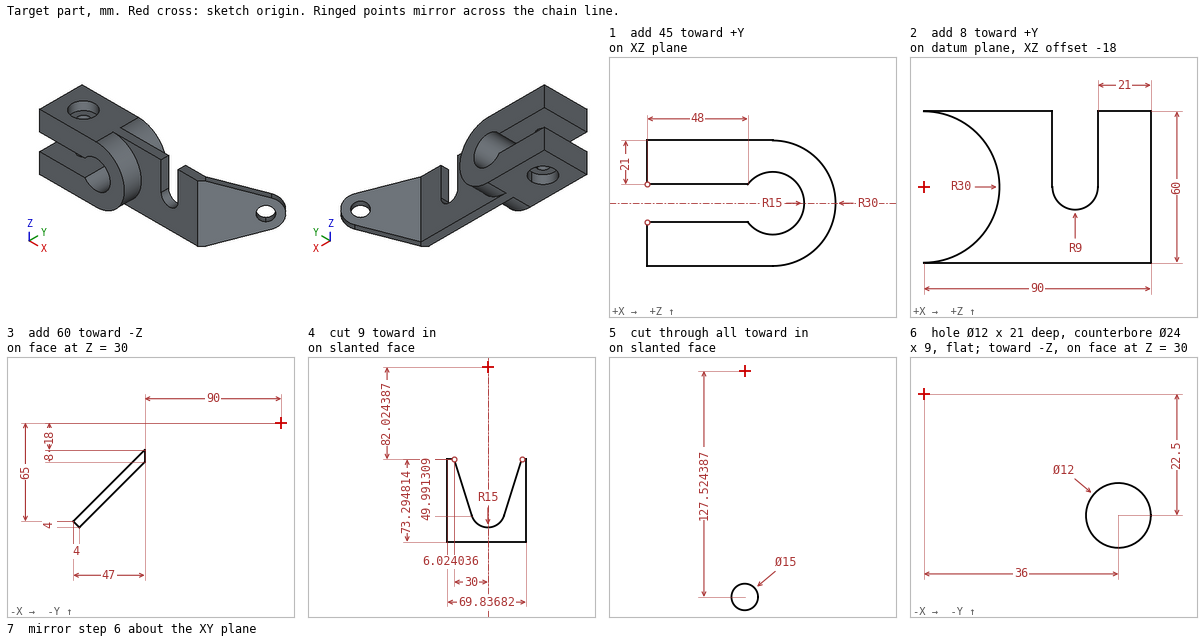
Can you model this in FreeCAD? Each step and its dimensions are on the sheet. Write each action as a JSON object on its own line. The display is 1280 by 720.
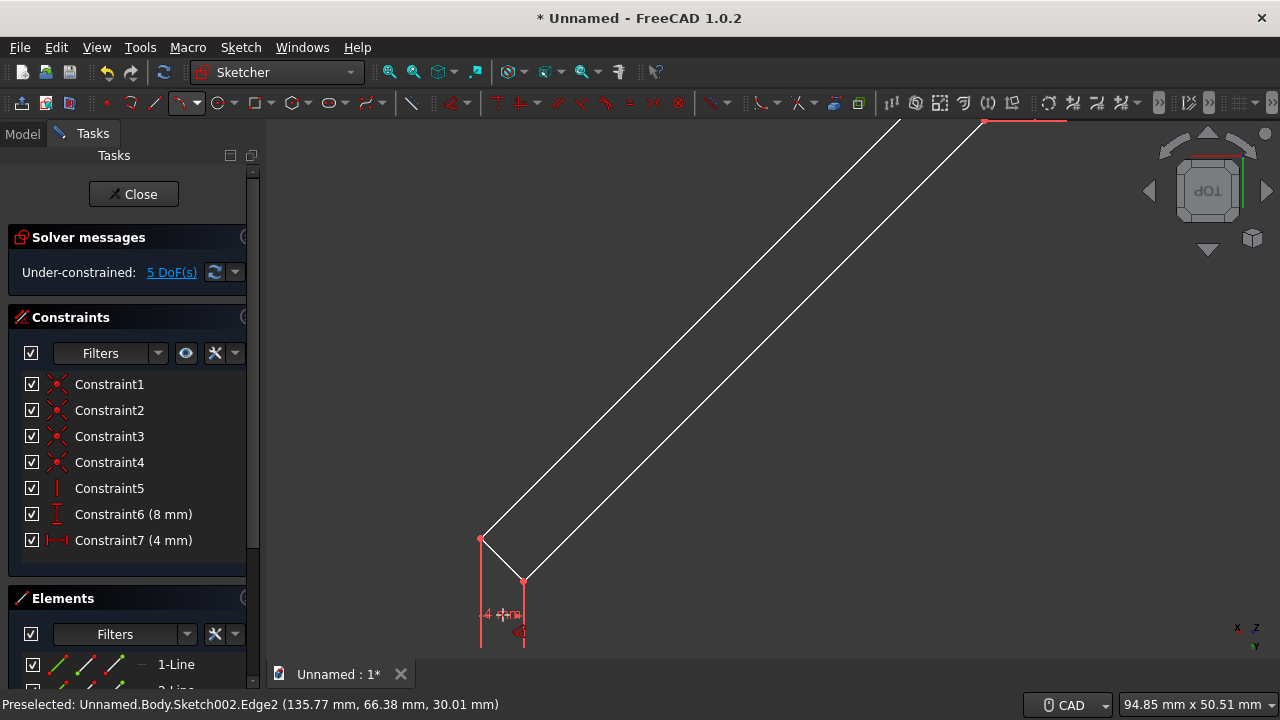
{"action": "left_click", "coordinate": [494, 551]}
{"action": "left_click", "coordinate": [447, 560]}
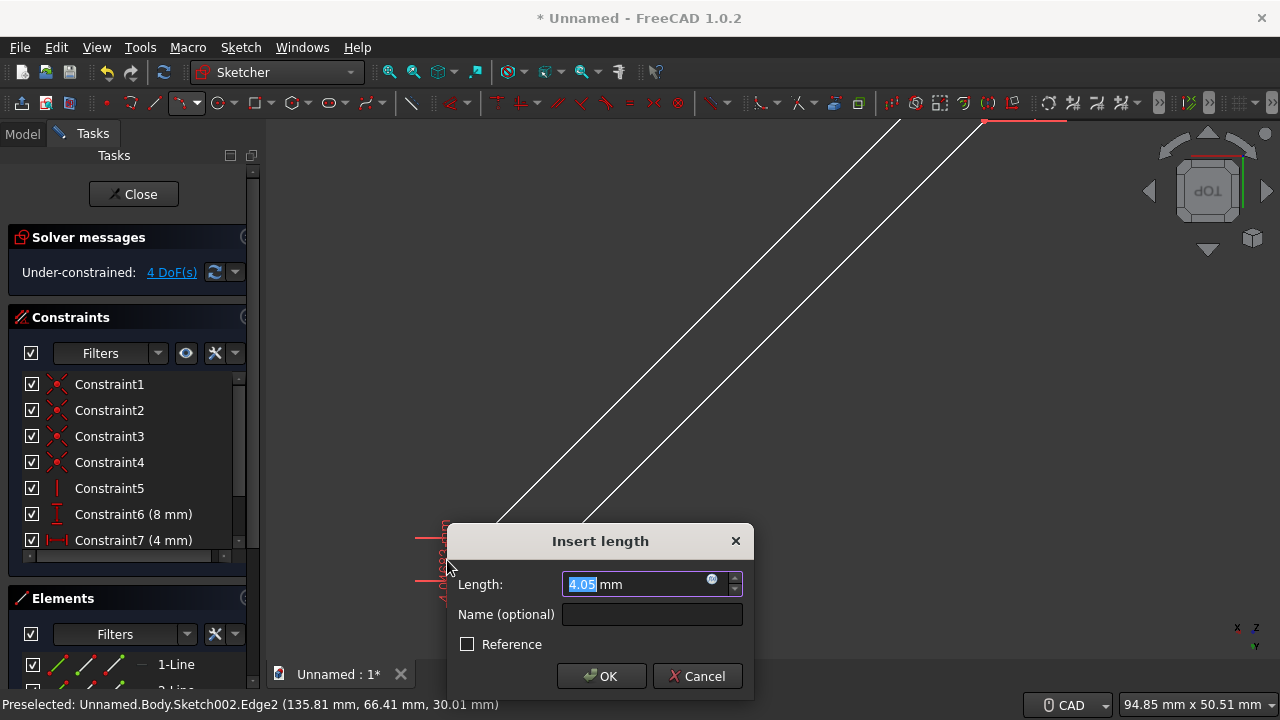
{"action": "type", "text": "4"}
{"action": "key", "text": "Return"}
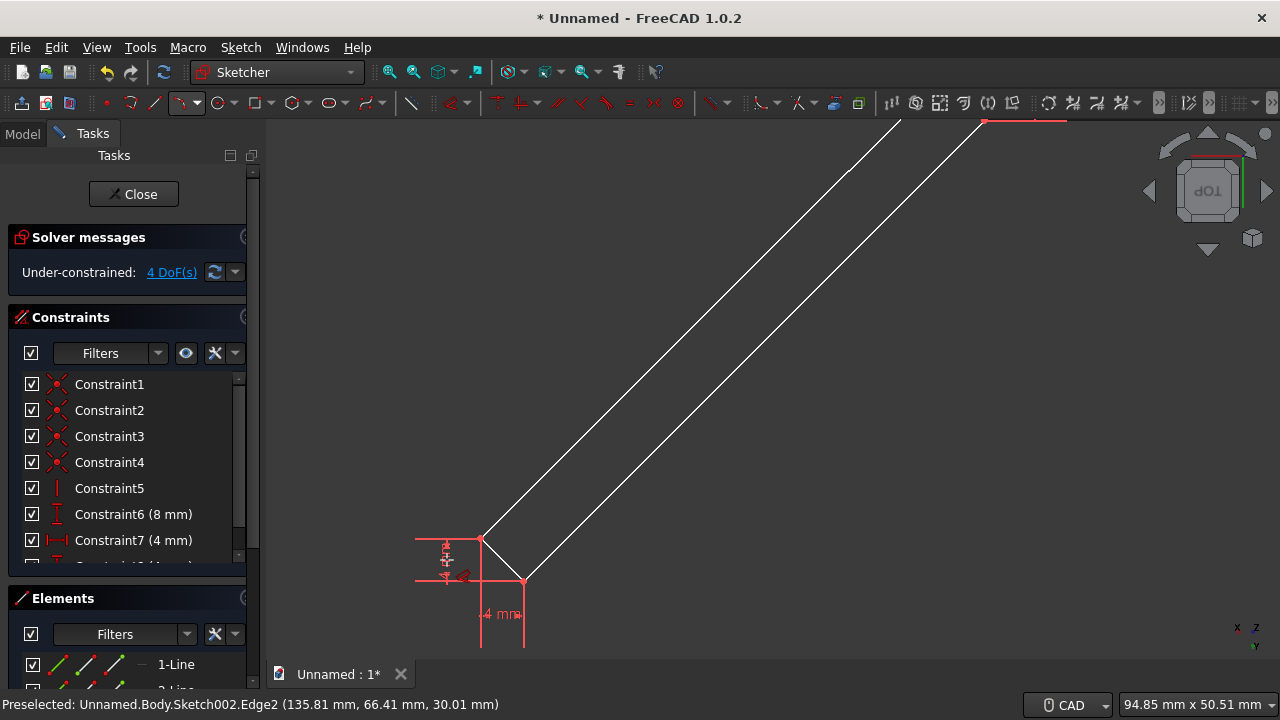
{"action": "scroll", "coordinate": [647, 556], "scroll_direction": "down", "scroll_amount": 2}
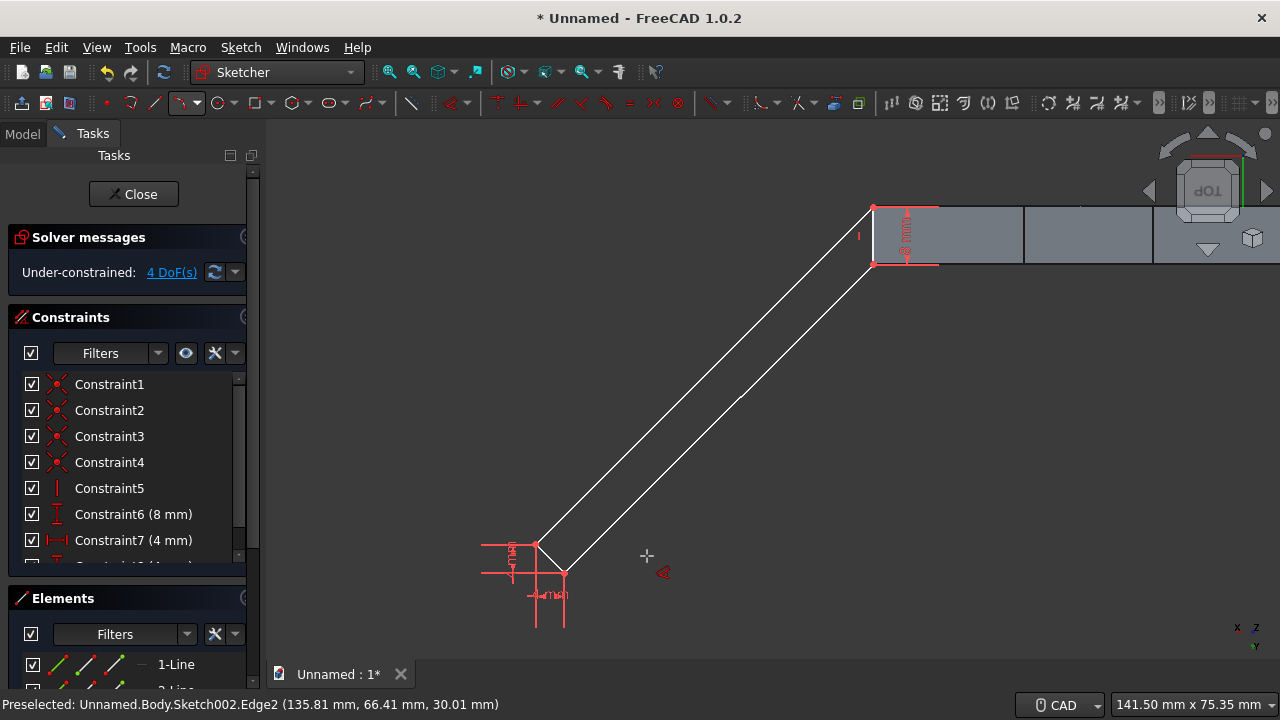
{"action": "left_click", "coordinate": [873, 207]}
{"action": "left_click", "coordinate": [994, 241]}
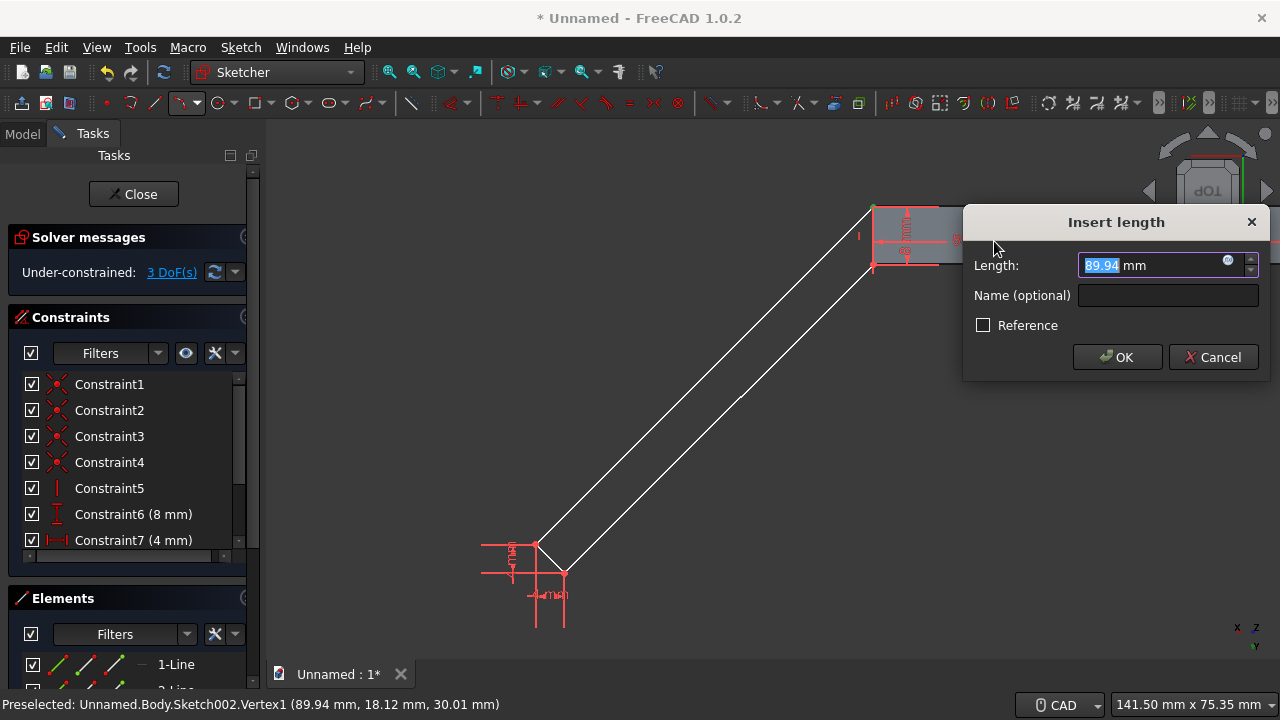
{"action": "type", "text": "90"}
{"action": "key", "text": "Return"}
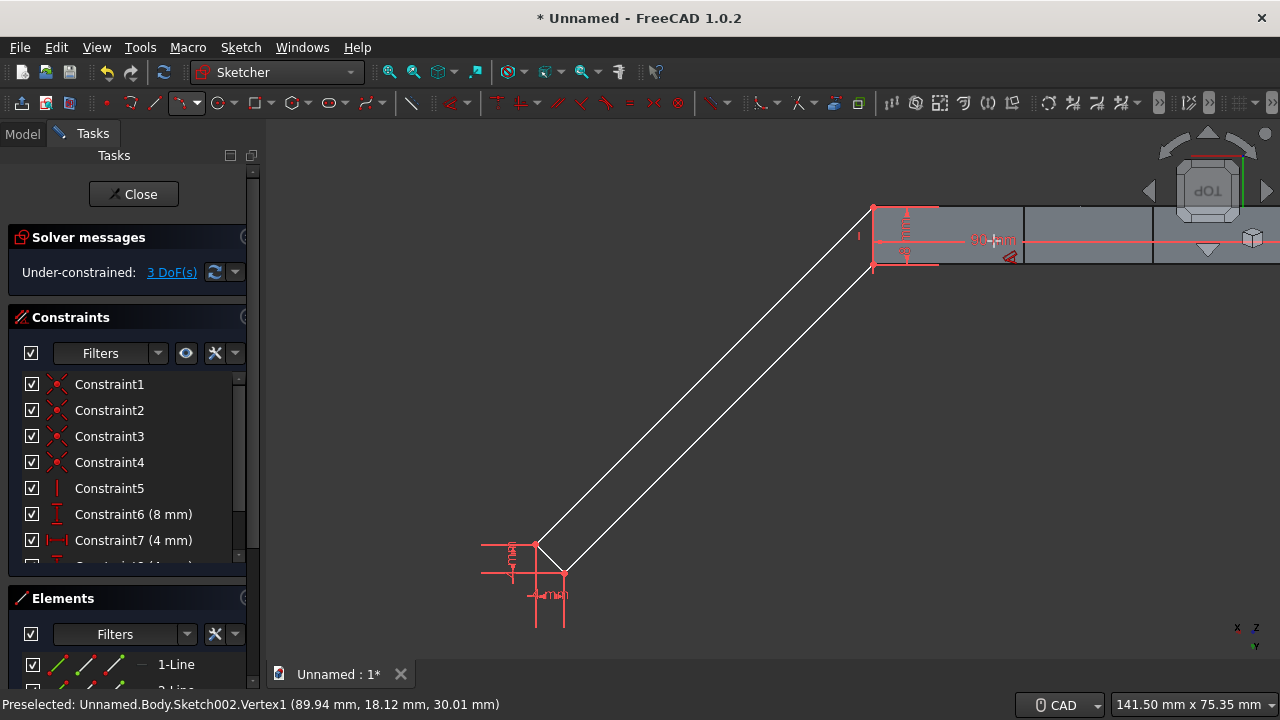
{"action": "left_click", "coordinate": [873, 207]}
{"action": "left_click", "coordinate": [839, 177]}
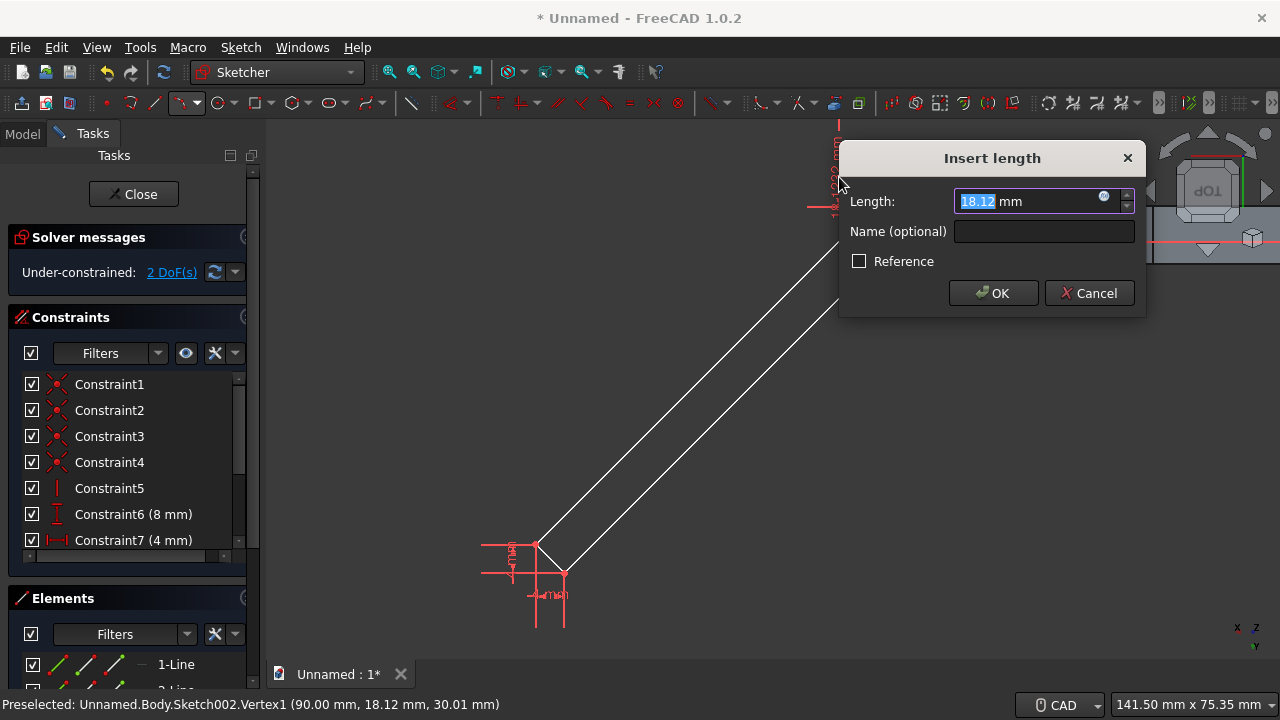
{"action": "type", "text": "18"}
{"action": "key", "text": "Return"}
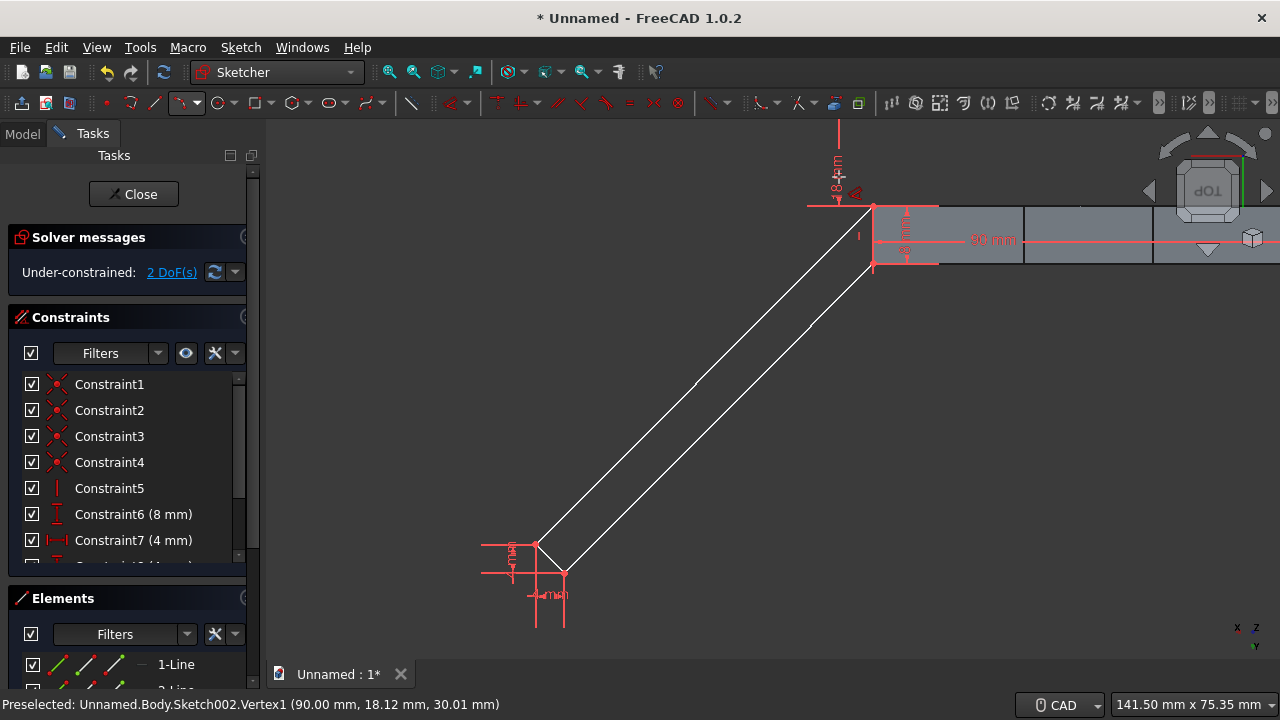
{"action": "left_click", "coordinate": [536, 545]}
{"action": "left_click", "coordinate": [502, 346]}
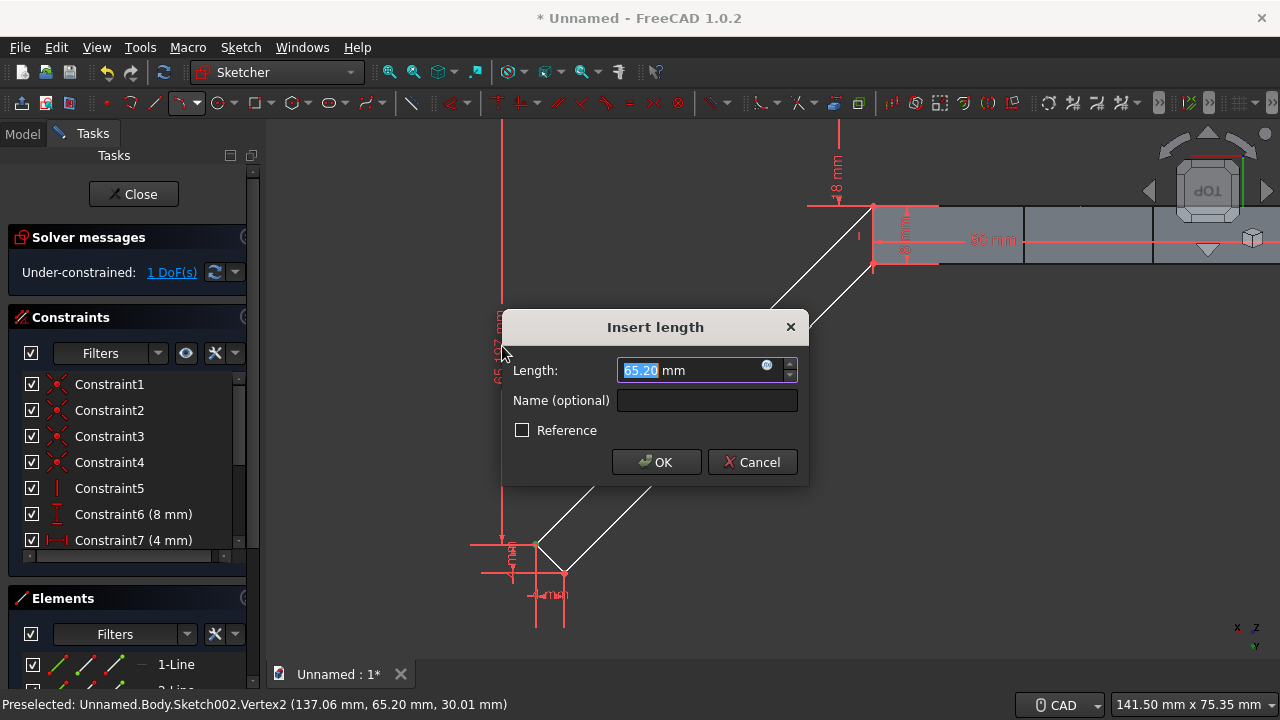
{"action": "type", "text": "65"}
{"action": "key", "text": "Return"}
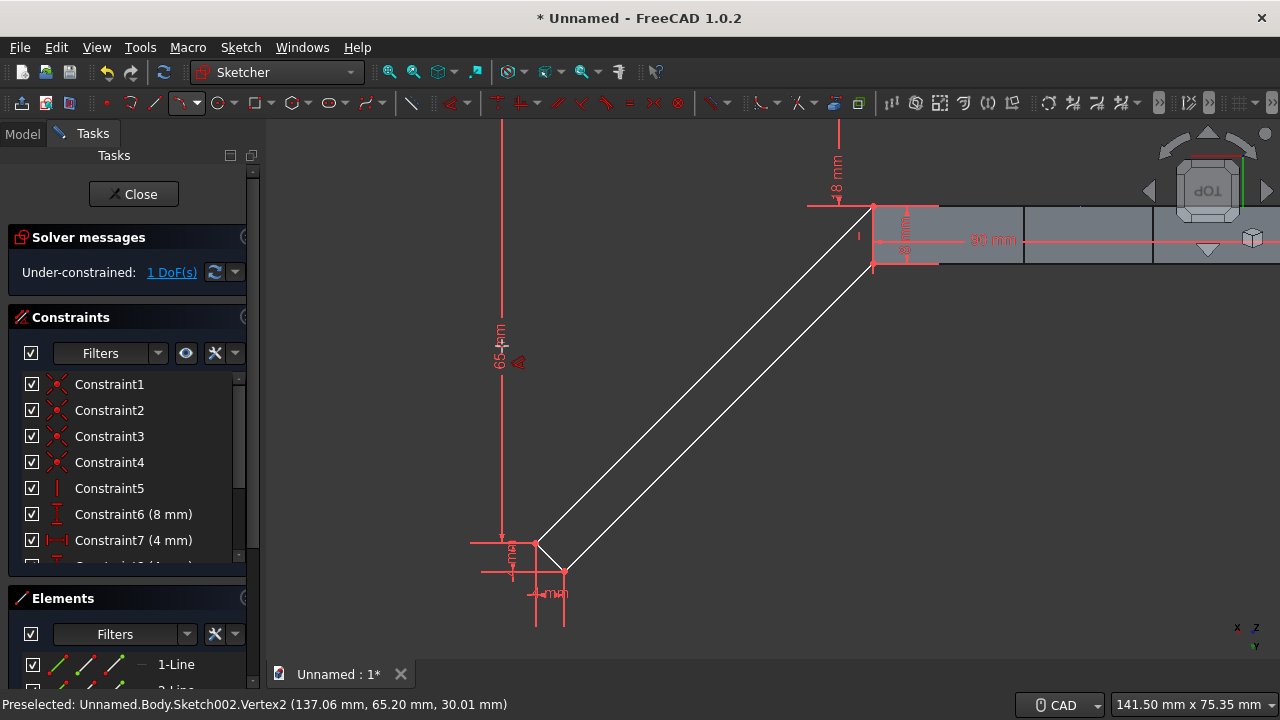
{"action": "left_click", "coordinate": [772, 307]}
{"action": "left_click", "coordinate": [704, 172]}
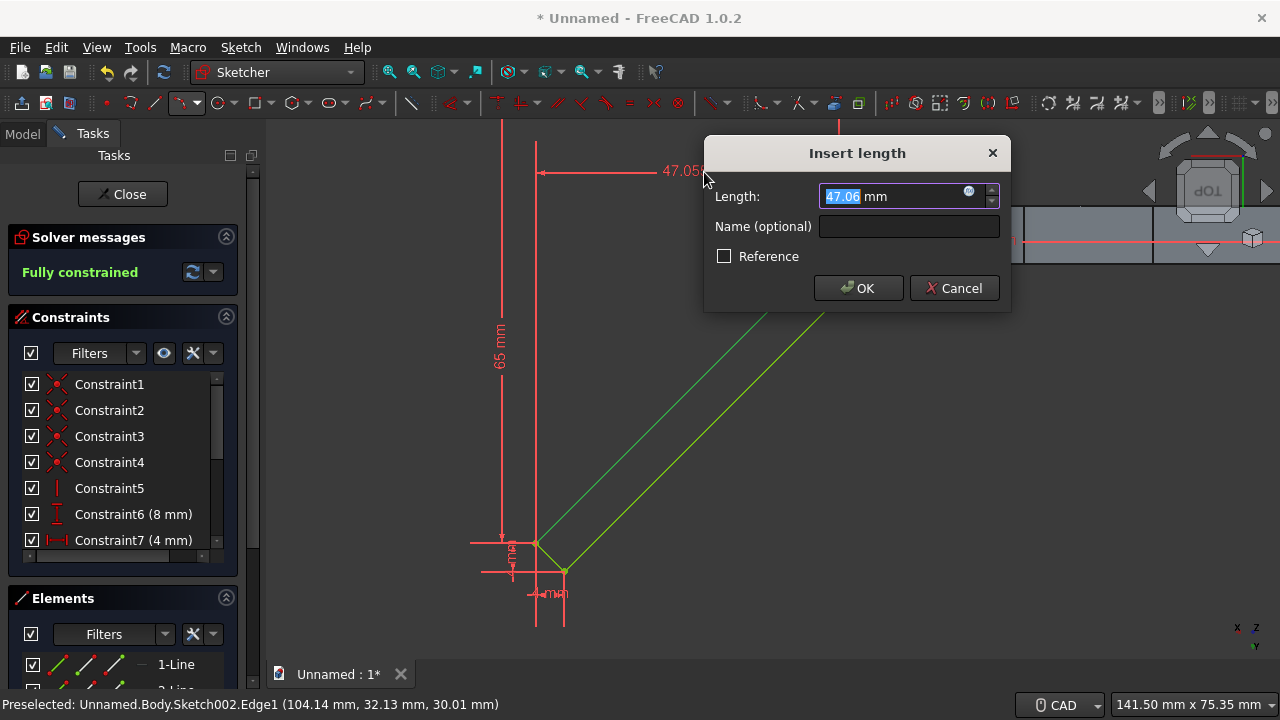
{"action": "type", "text": "47"}
{"action": "key", "text": "Return"}
{"action": "key", "text": "Escape"}